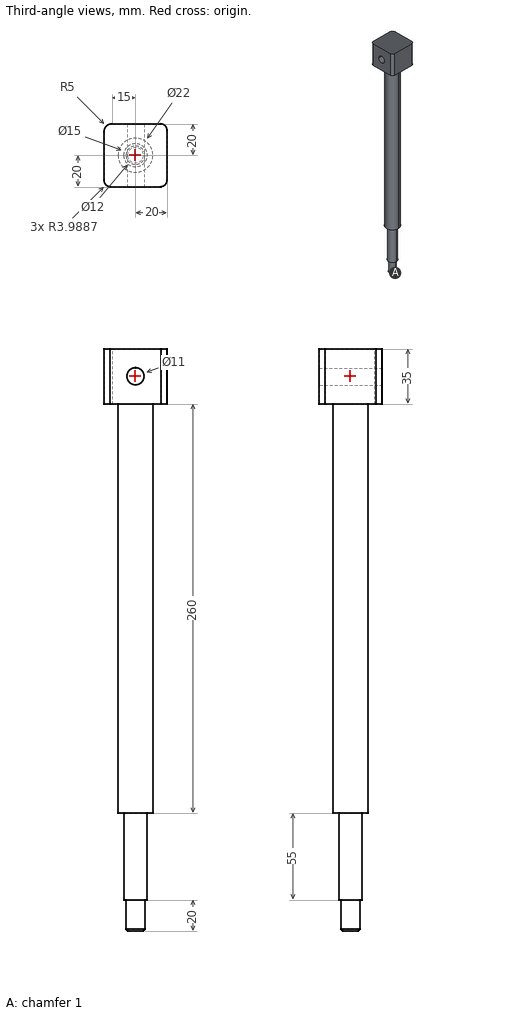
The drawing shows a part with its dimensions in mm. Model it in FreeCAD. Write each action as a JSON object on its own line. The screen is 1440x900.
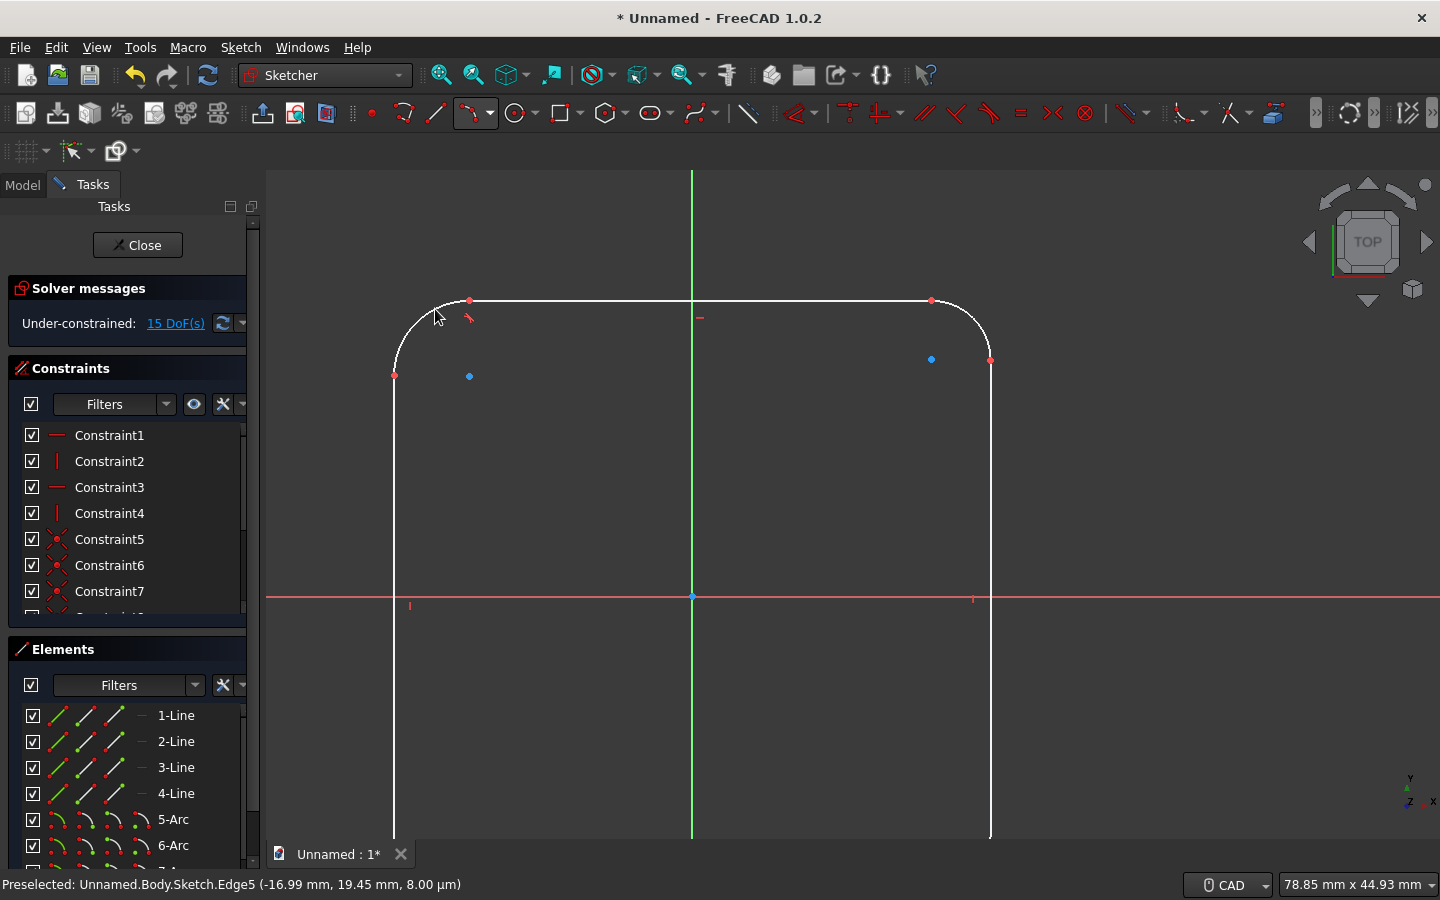
{"action": "left_click", "coordinate": [793, 301]}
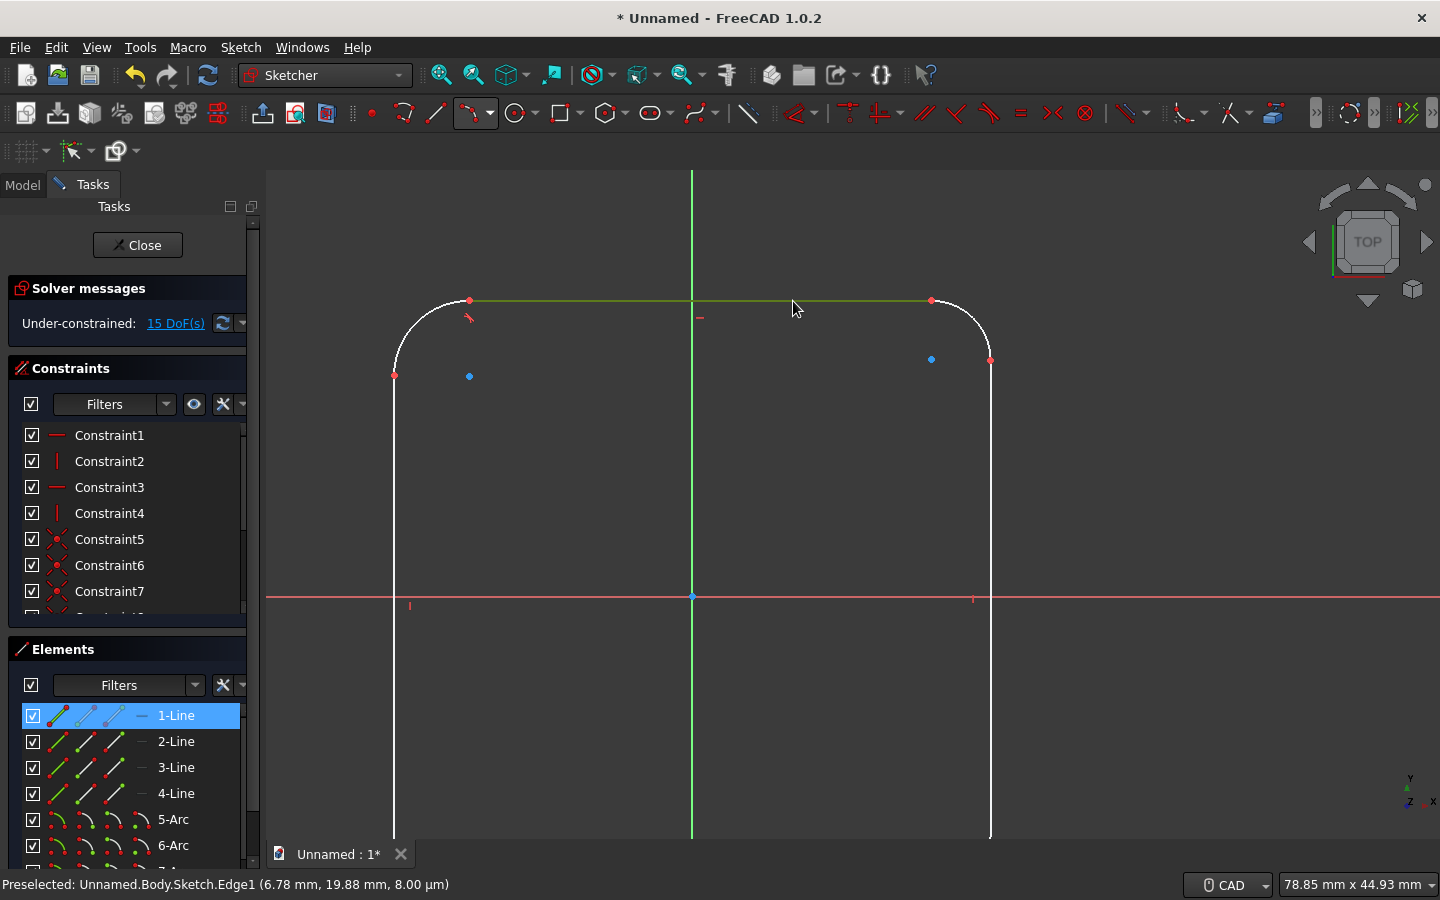
{"action": "left_click", "coordinate": [984, 333]}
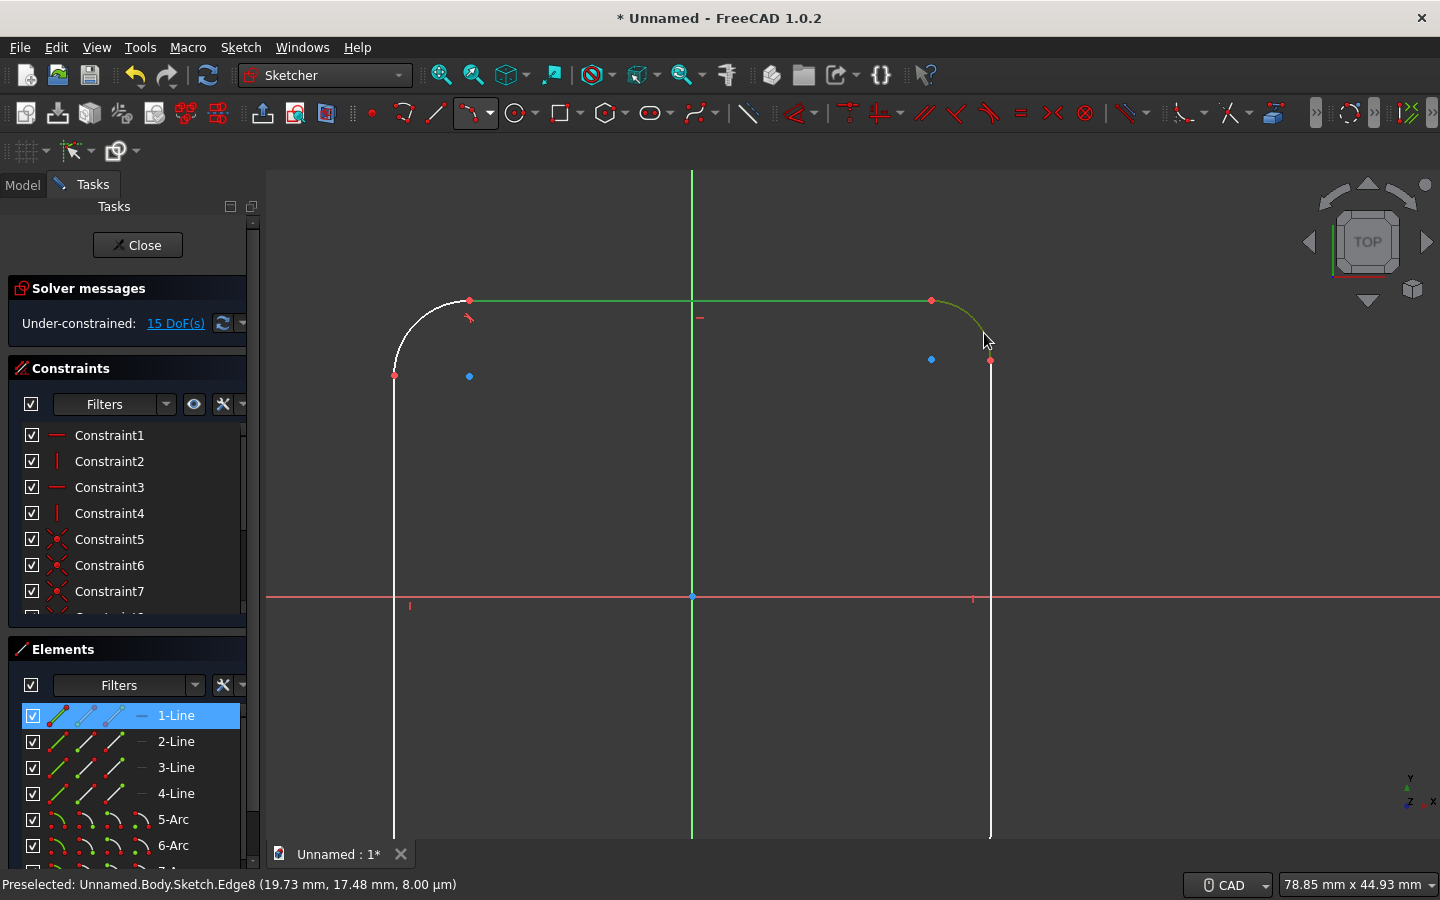
{"action": "left_click", "coordinate": [990, 114]}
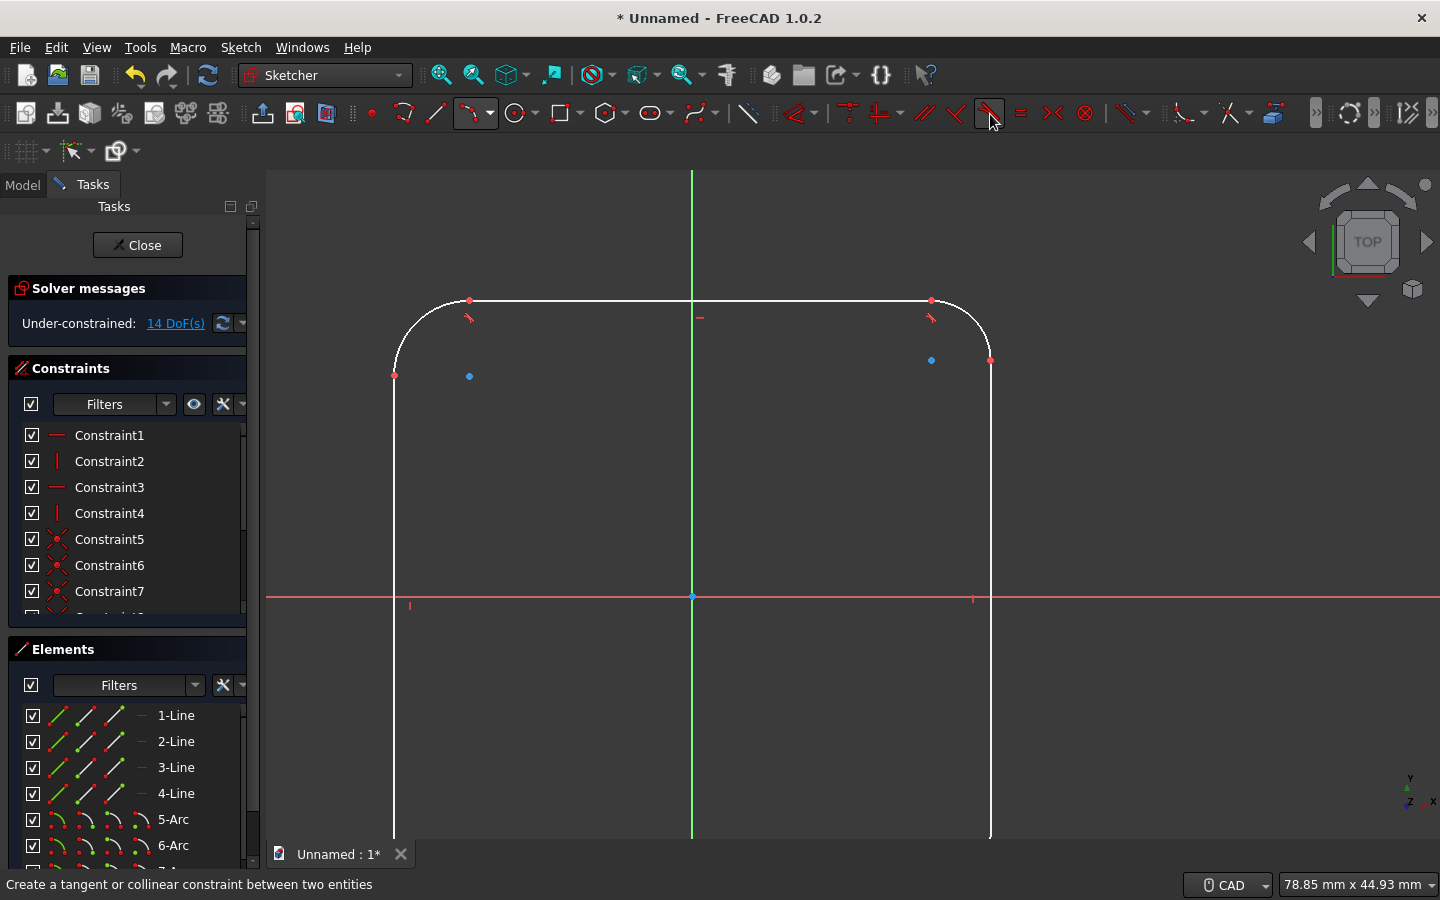
{"action": "left_click", "coordinate": [394, 514]}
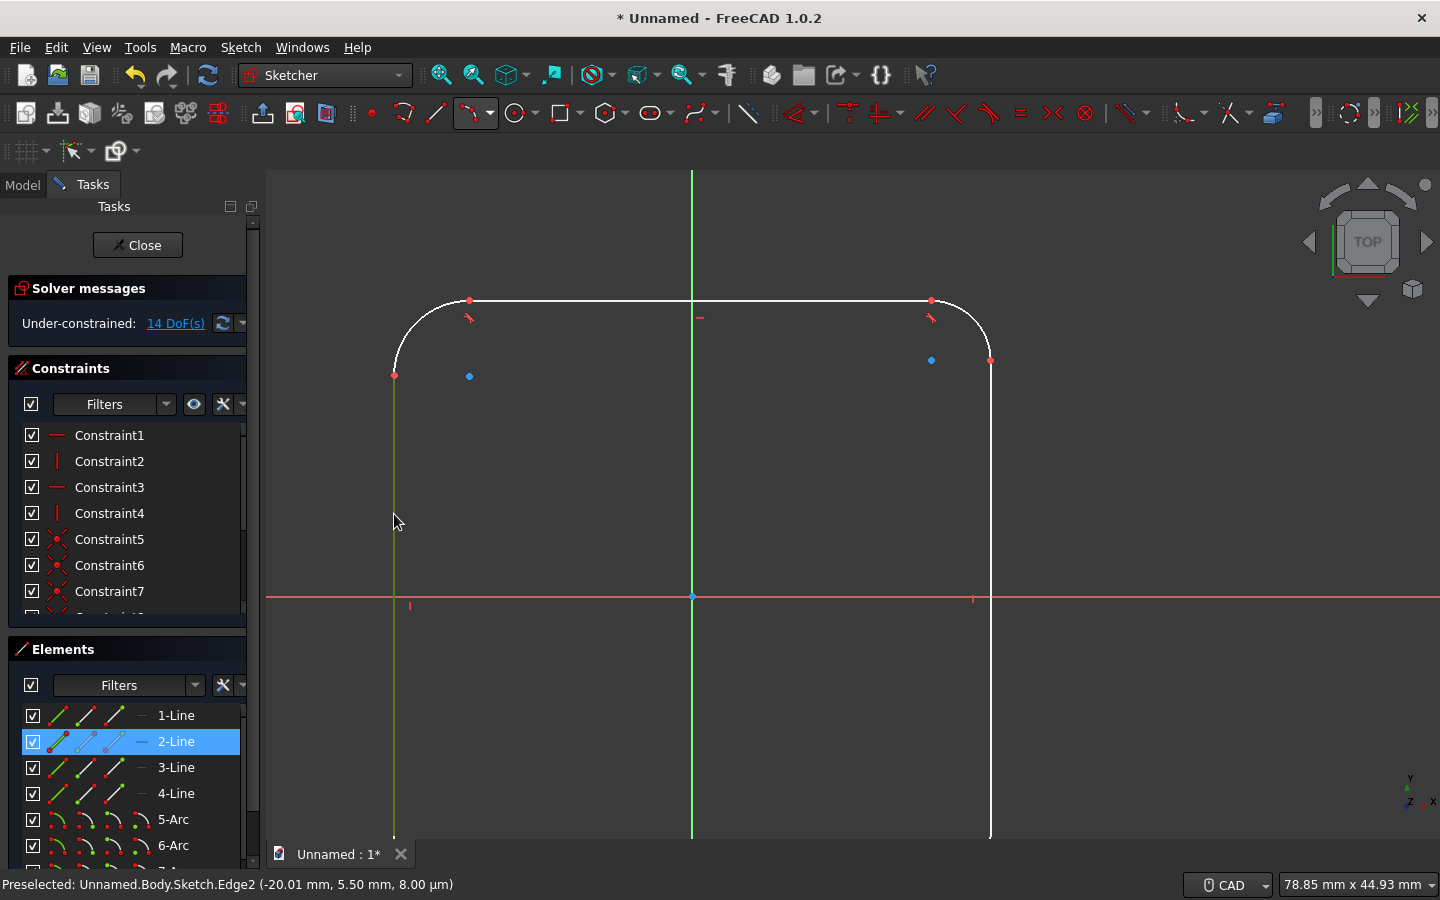
{"action": "left_click", "coordinate": [436, 309]}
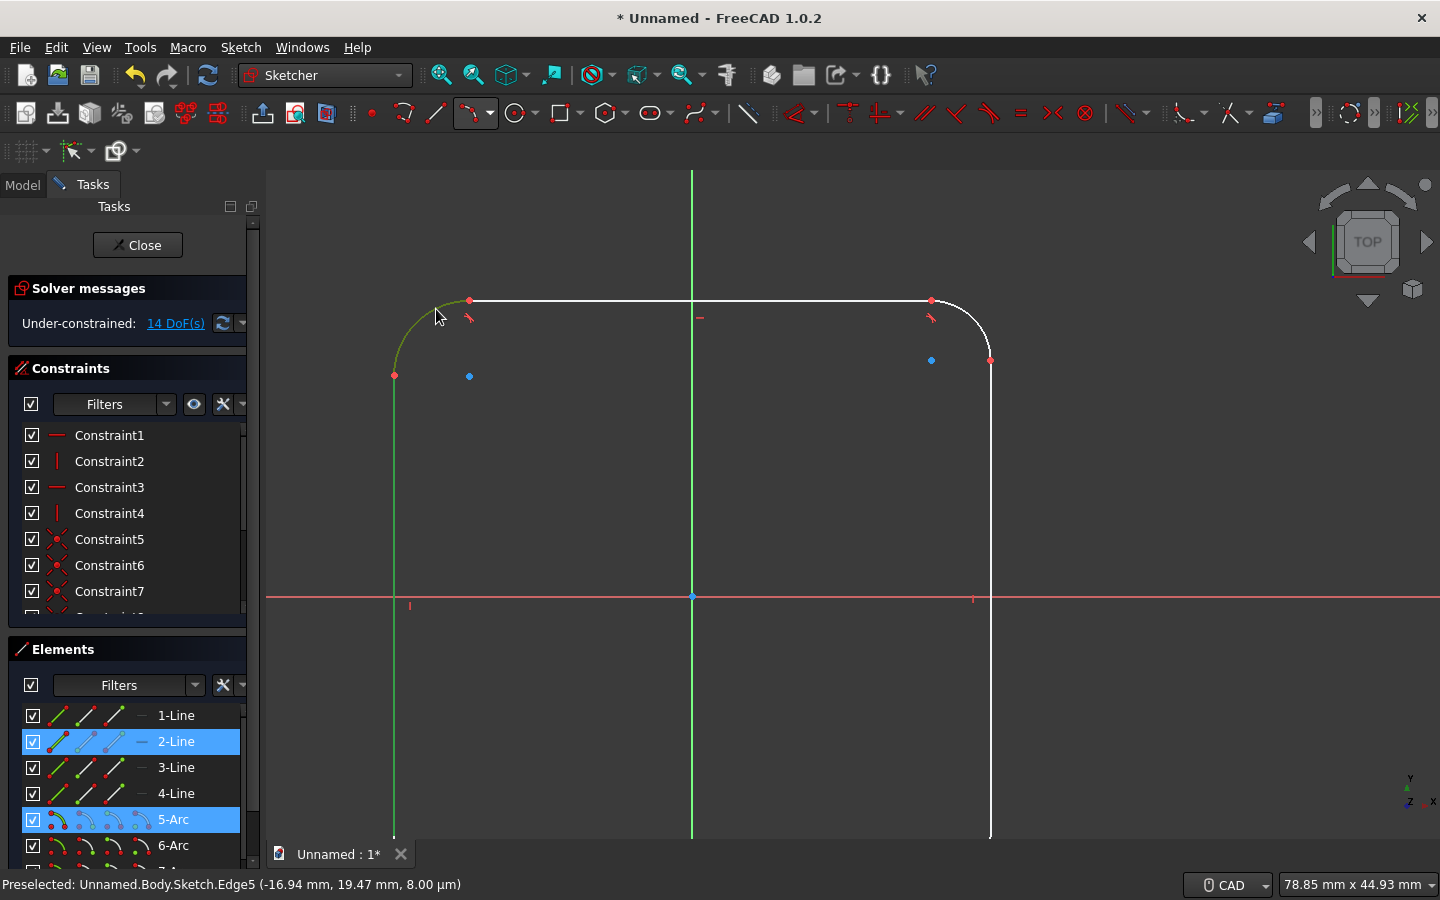
{"action": "left_click", "coordinate": [990, 114]}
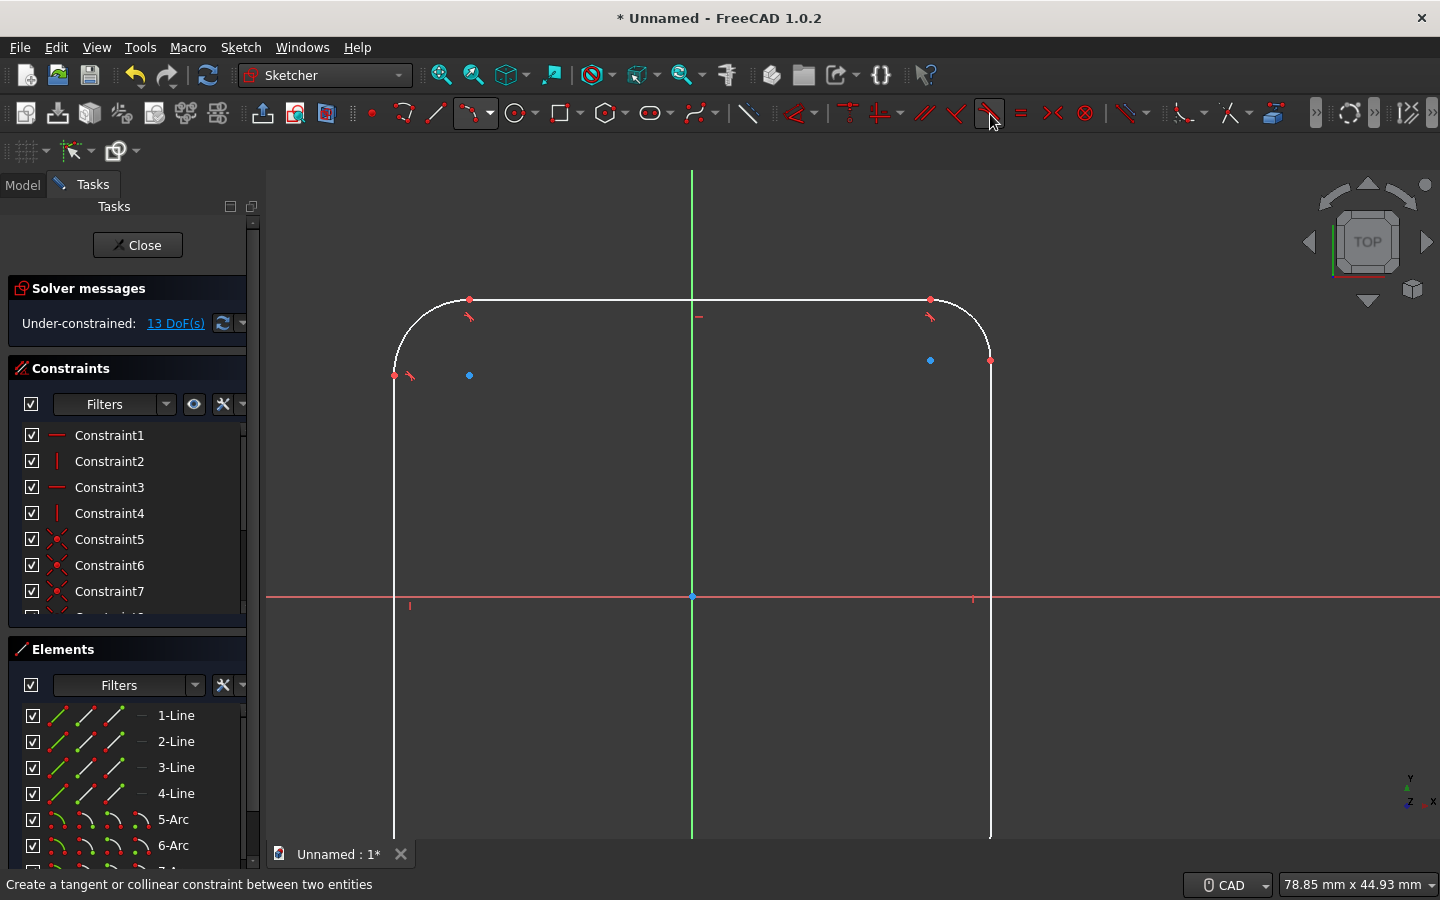
{"action": "left_click", "coordinate": [394, 514]}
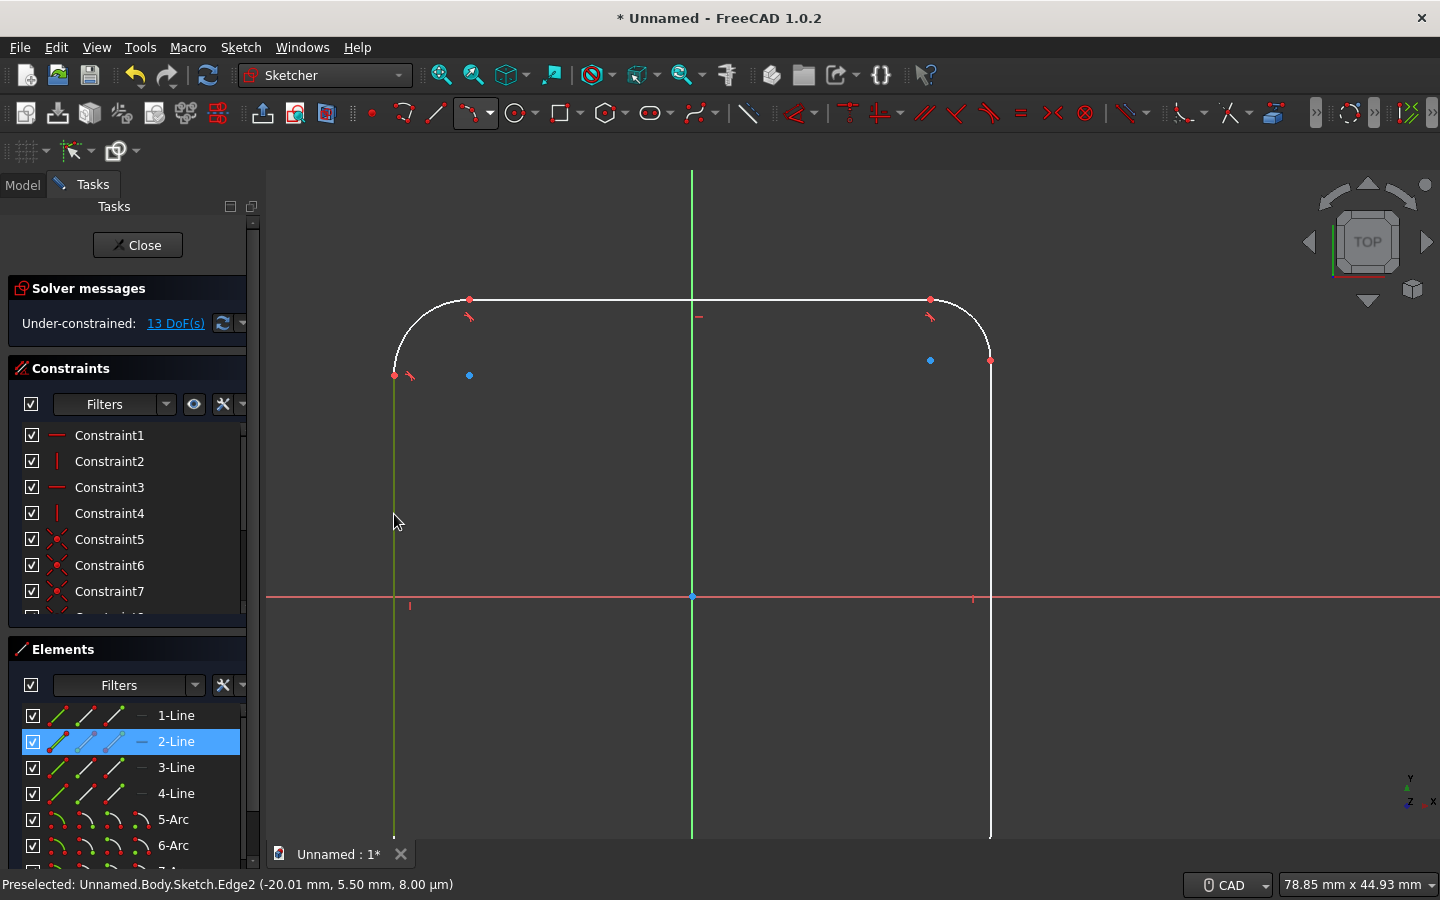
{"action": "scroll", "coordinate": [972, 317], "scroll_direction": "down", "scroll_amount": 2}